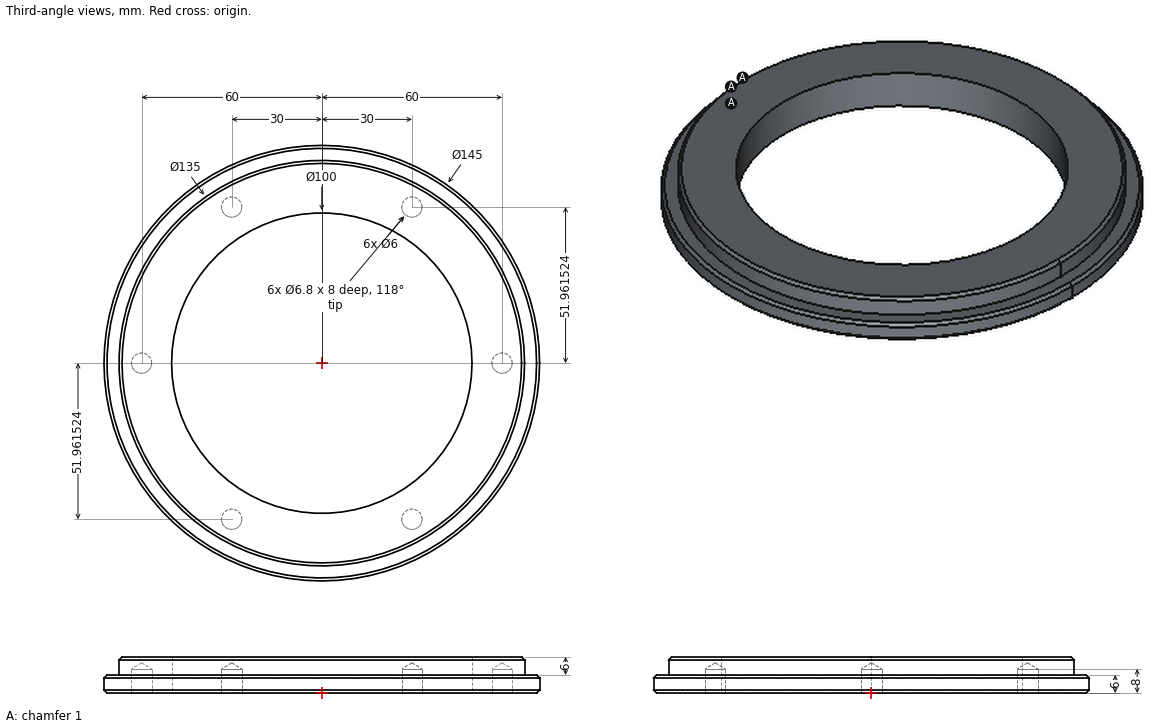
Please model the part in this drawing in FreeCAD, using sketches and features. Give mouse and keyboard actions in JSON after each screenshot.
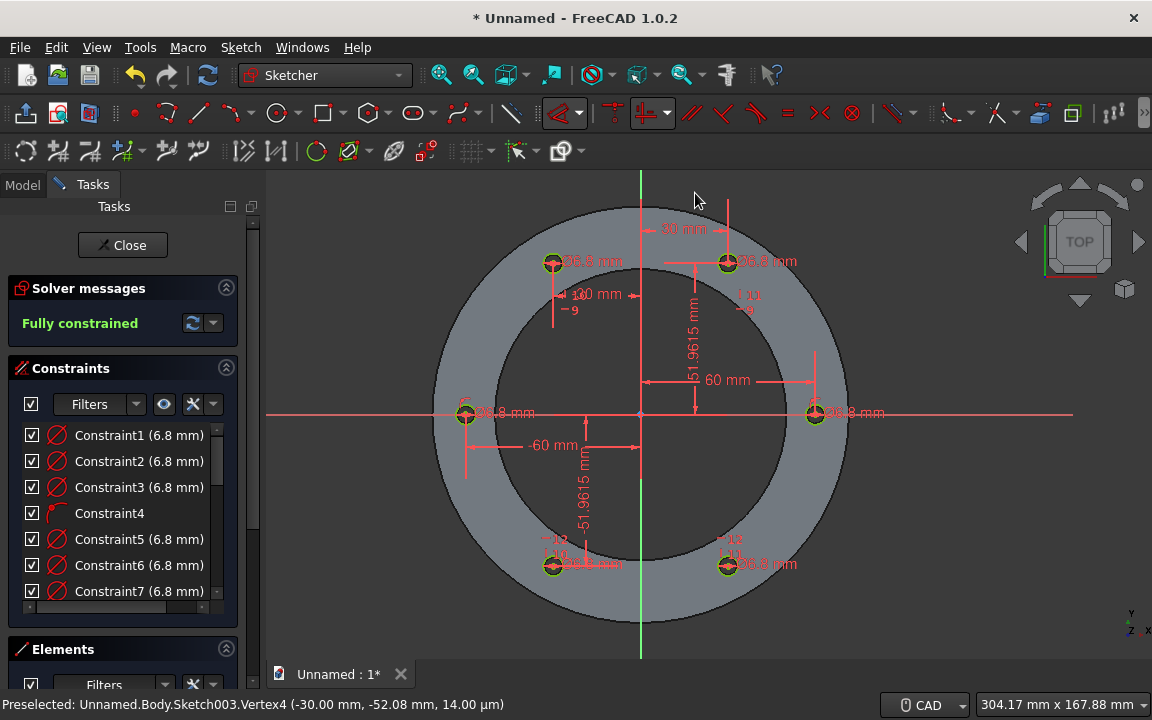
{"action": "left_click", "coordinate": [123, 245]}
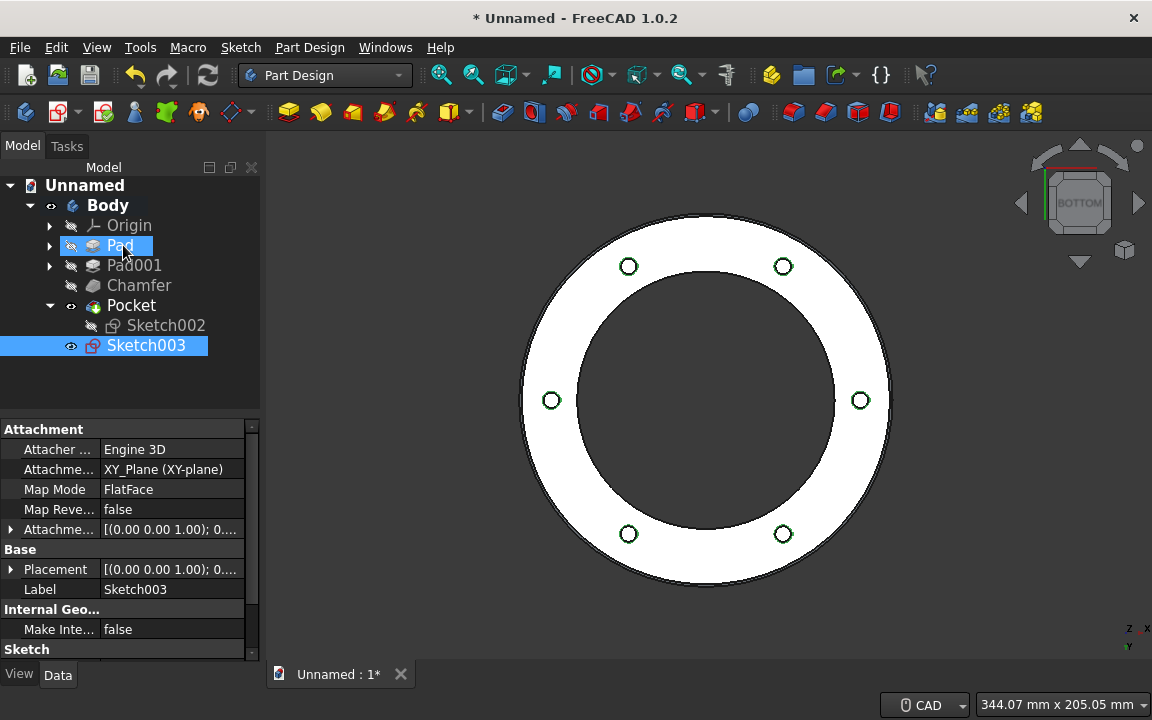
{"action": "left_click", "coordinate": [536, 112]}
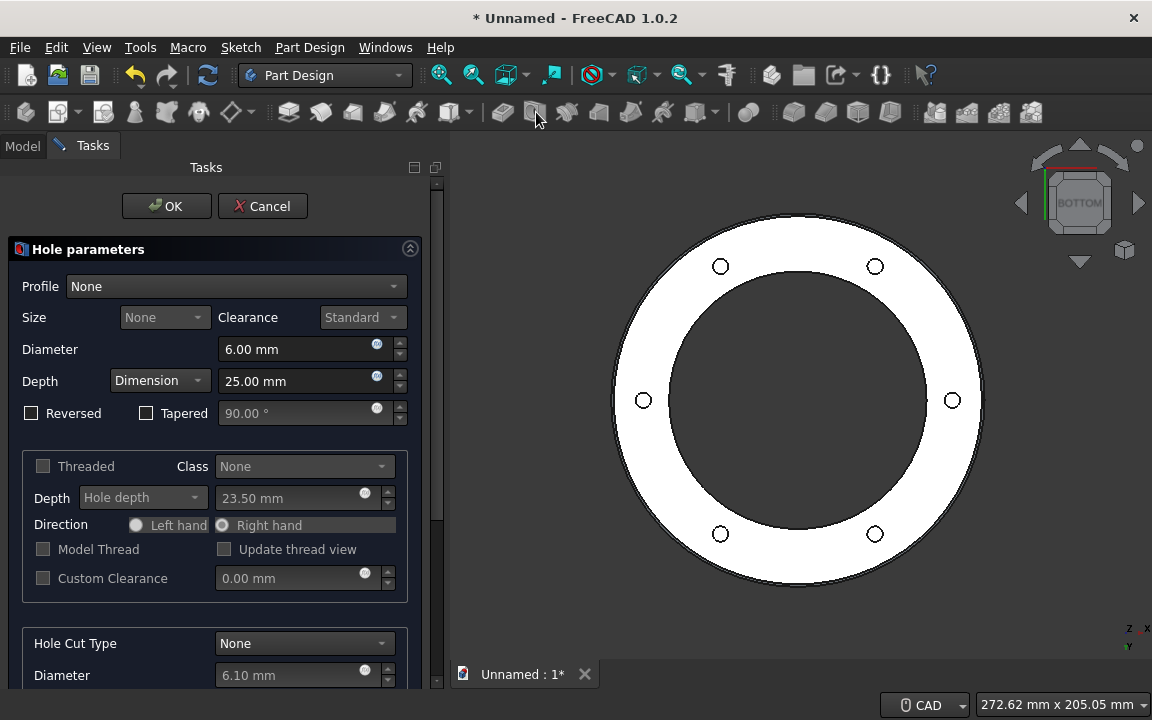
{"action": "triple_click", "coordinate": [305, 349]}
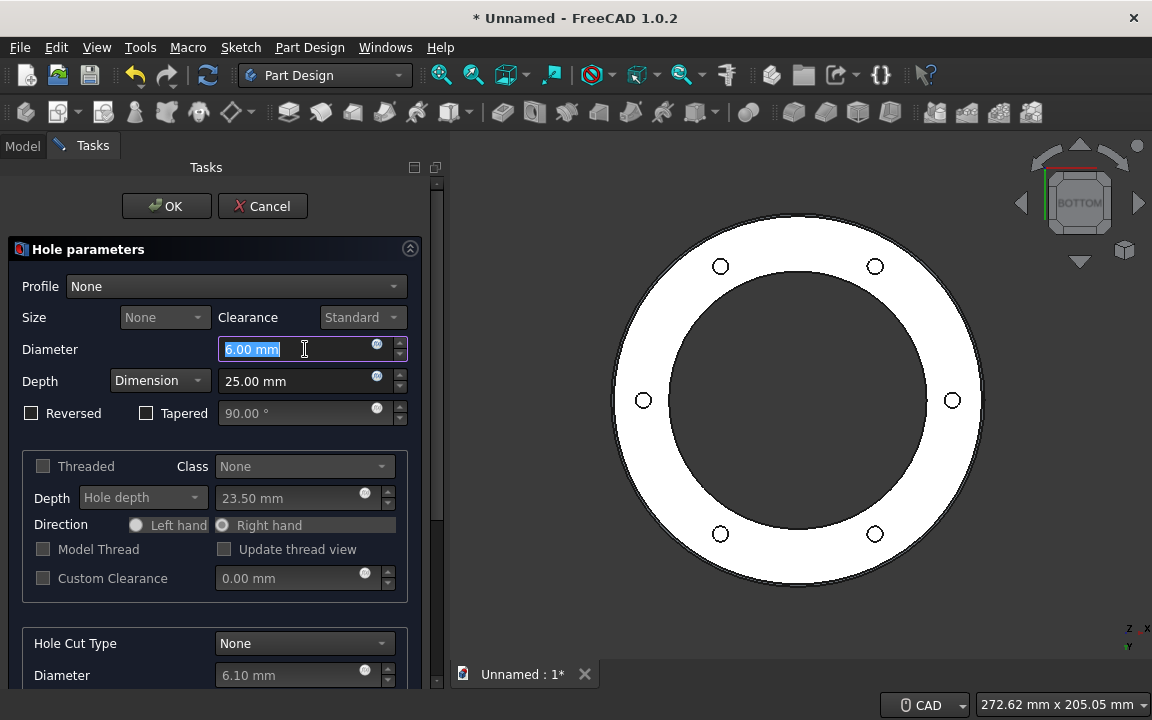
{"action": "type", "text": "6.8"}
{"action": "key", "text": "Tab"}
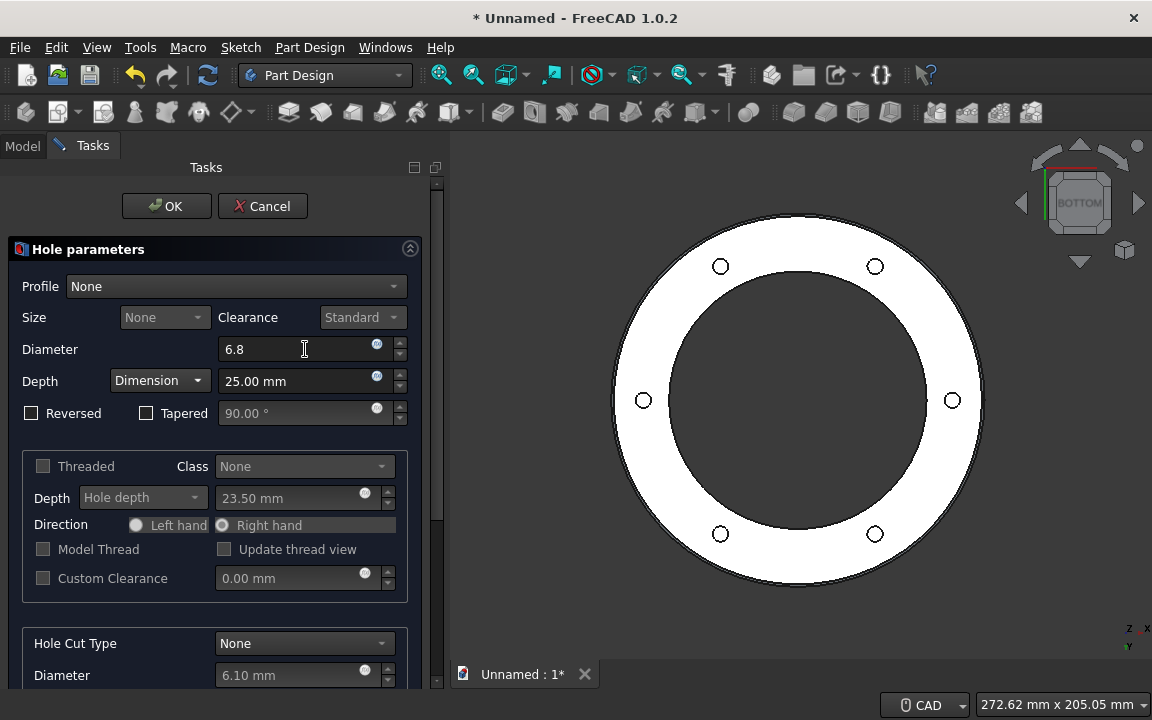
{"action": "triple_click", "coordinate": [305, 381]}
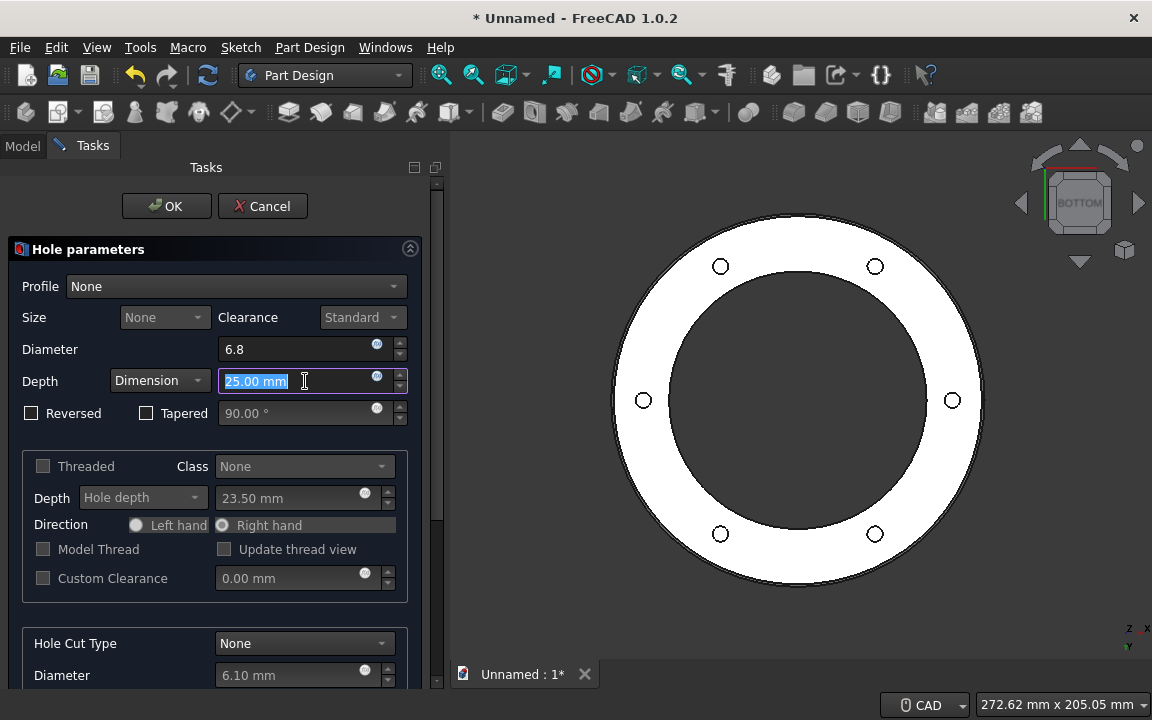
{"action": "type", "text": "8"}
{"action": "key", "text": "Tab"}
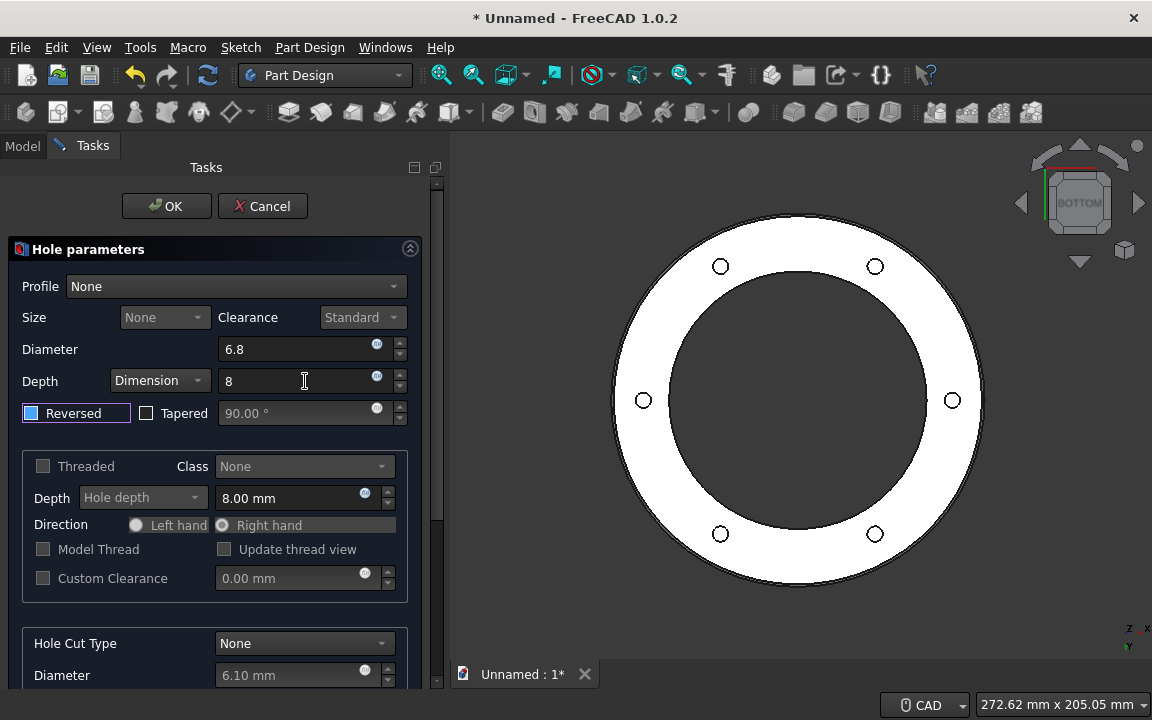
{"action": "left_click", "coordinate": [30, 413]}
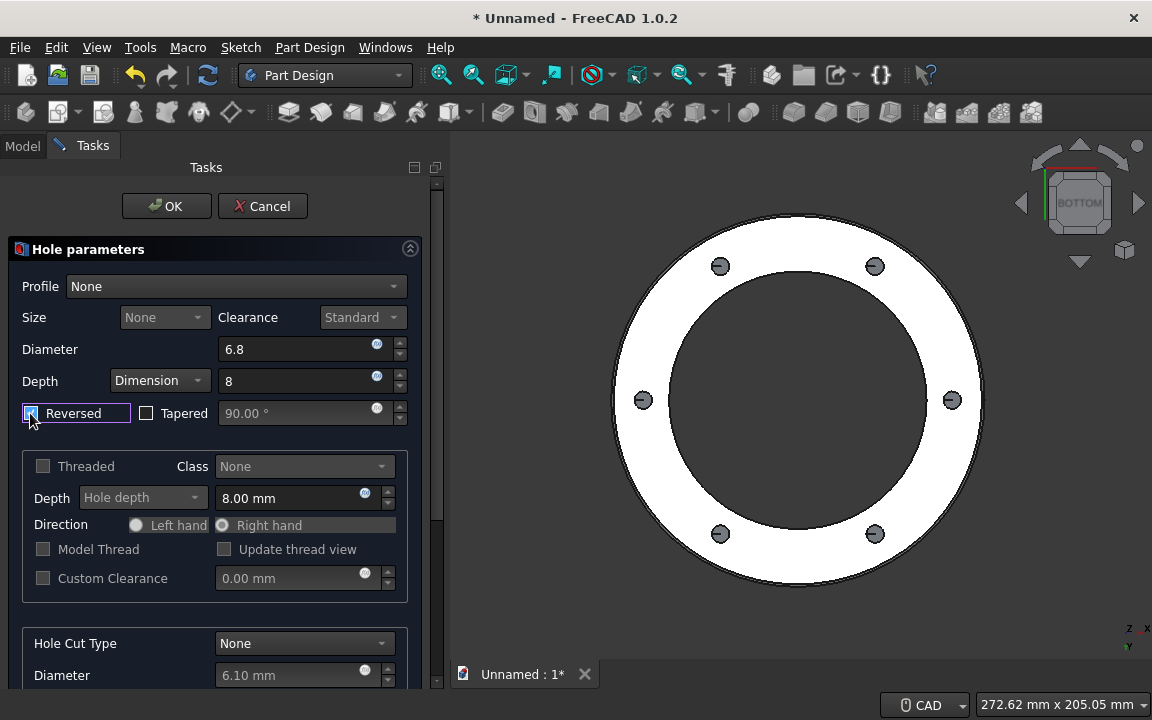
{"action": "left_click", "coordinate": [167, 206]}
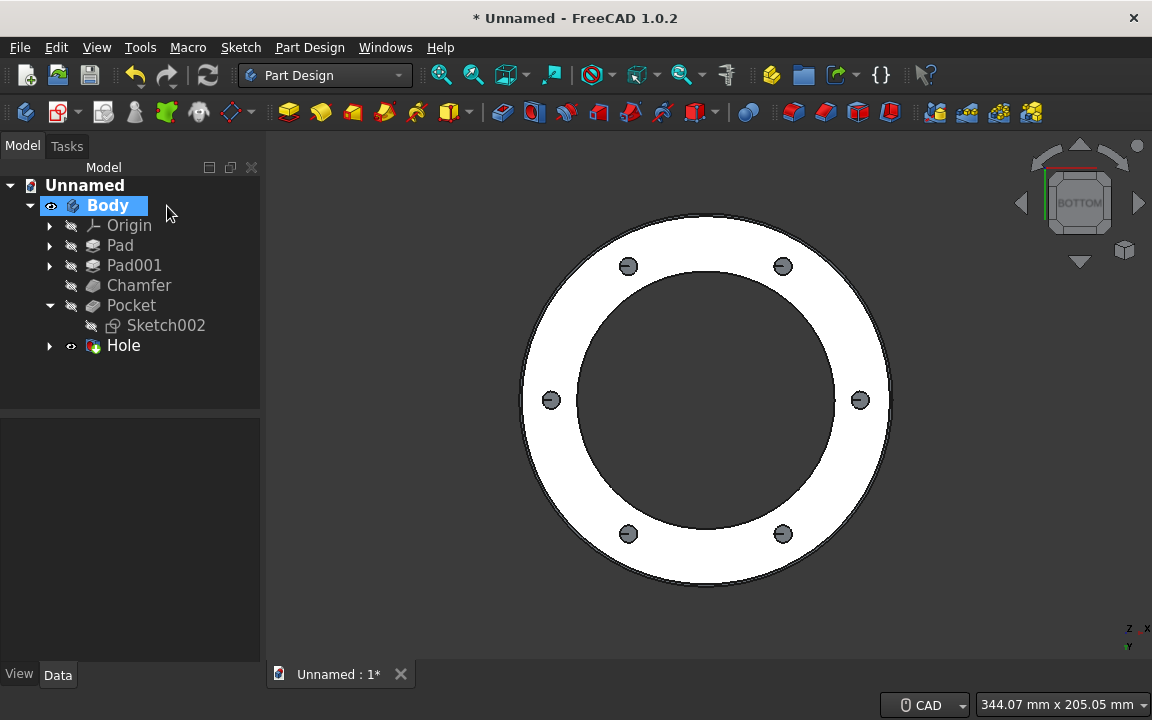
{"action": "key", "text": "0"}